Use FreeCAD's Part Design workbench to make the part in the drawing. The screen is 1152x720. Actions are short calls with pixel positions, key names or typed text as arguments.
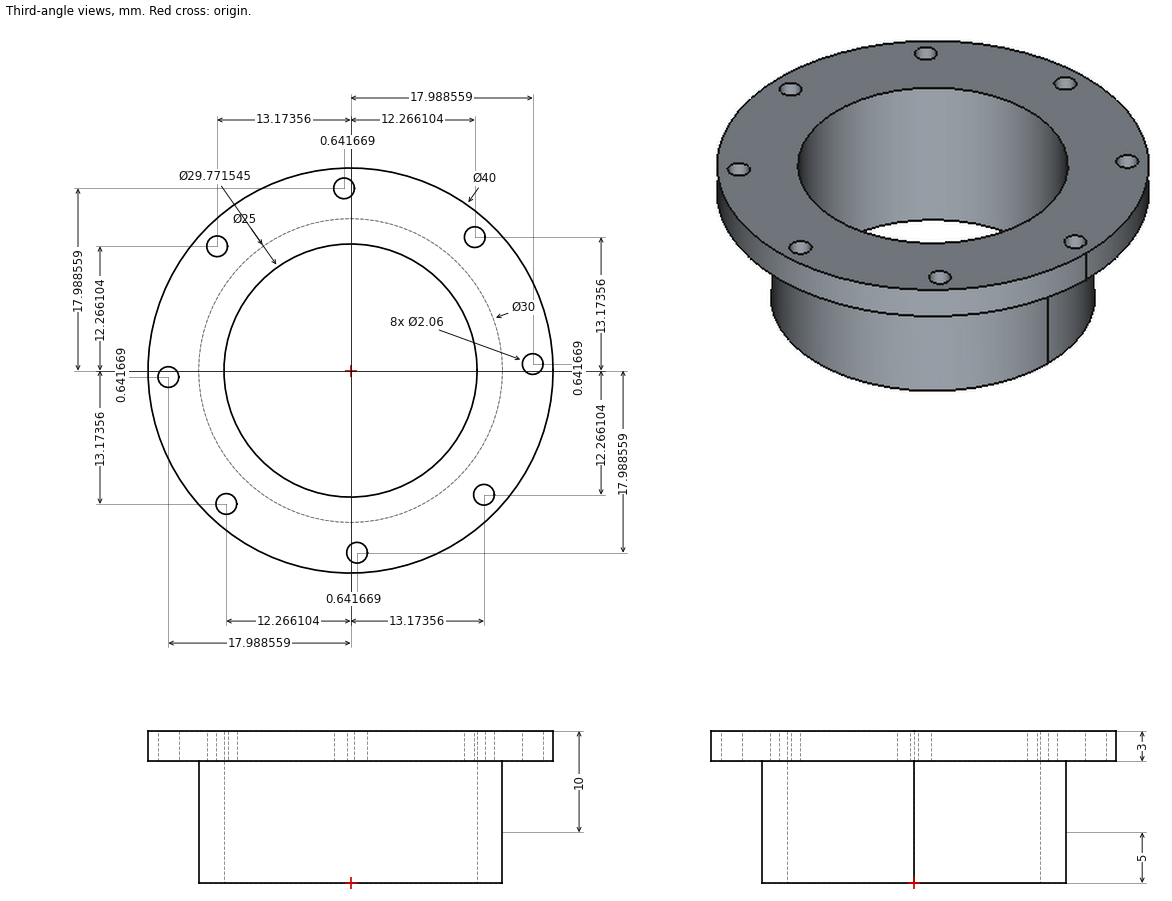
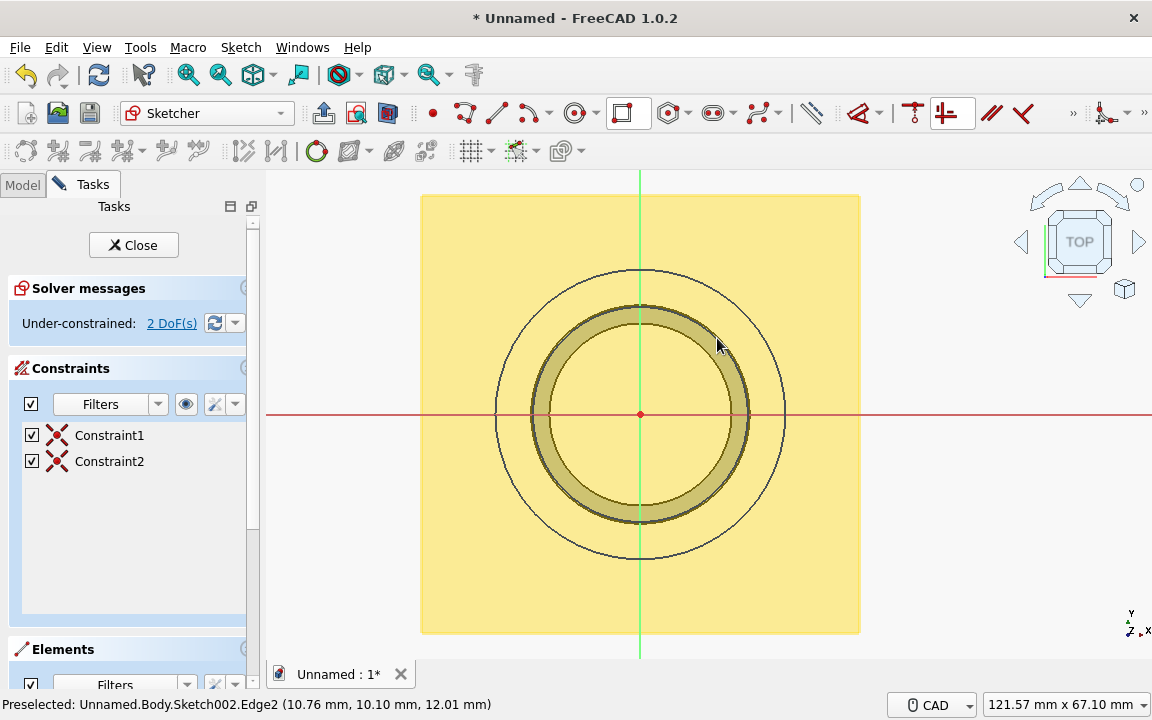
click(858, 114)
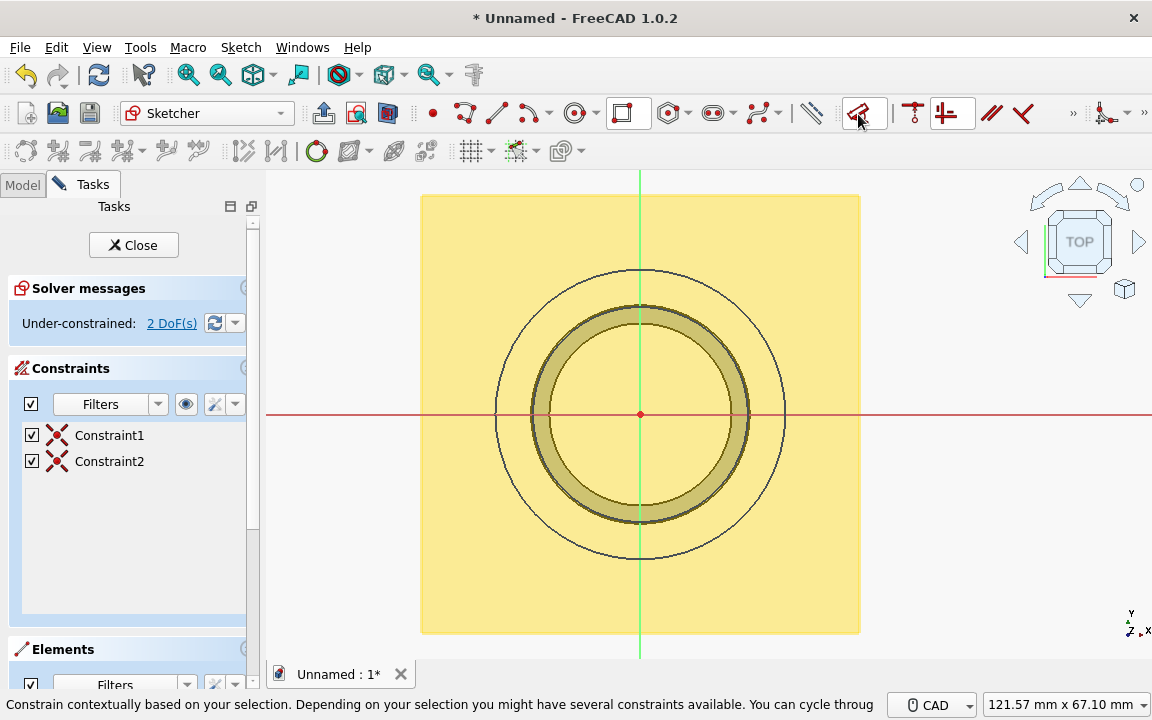
click(743, 312)
click(766, 289)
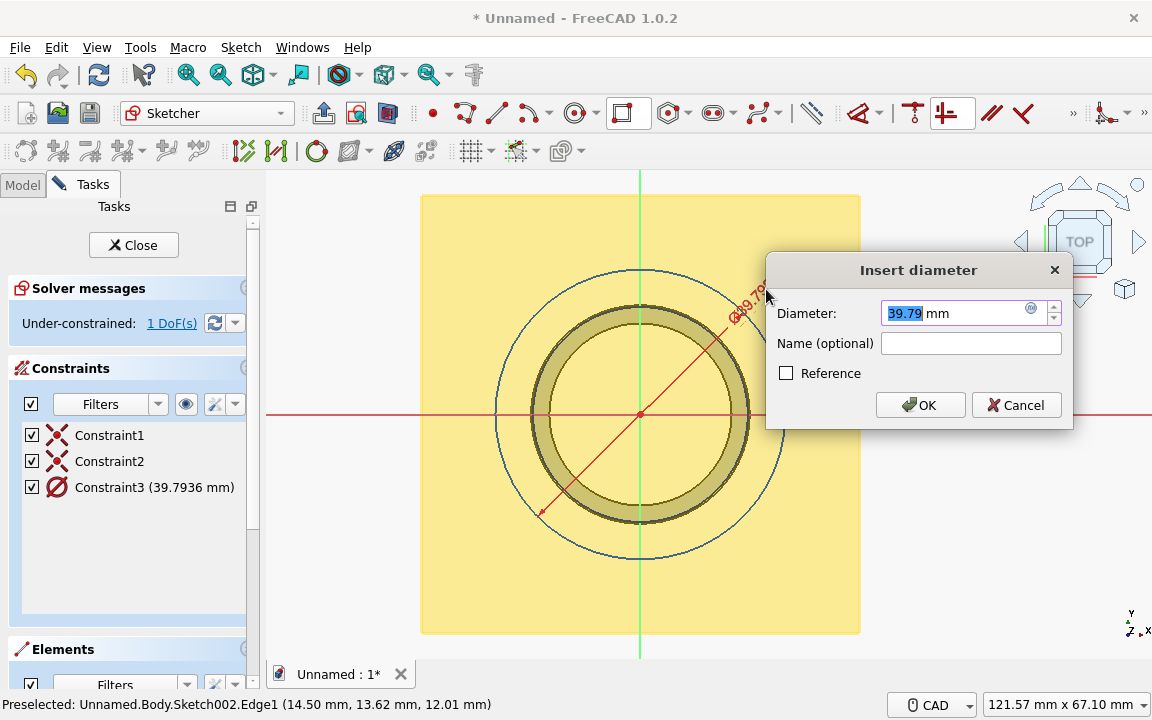
text(40)
key(Return)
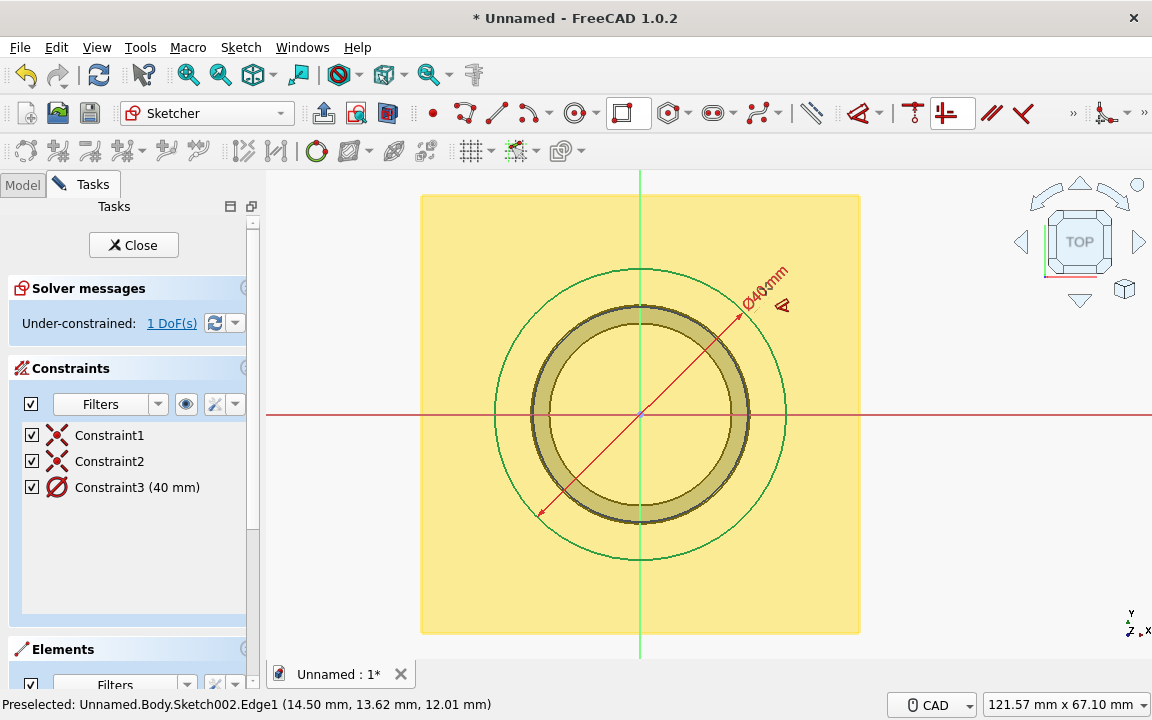
click(716, 338)
click(796, 368)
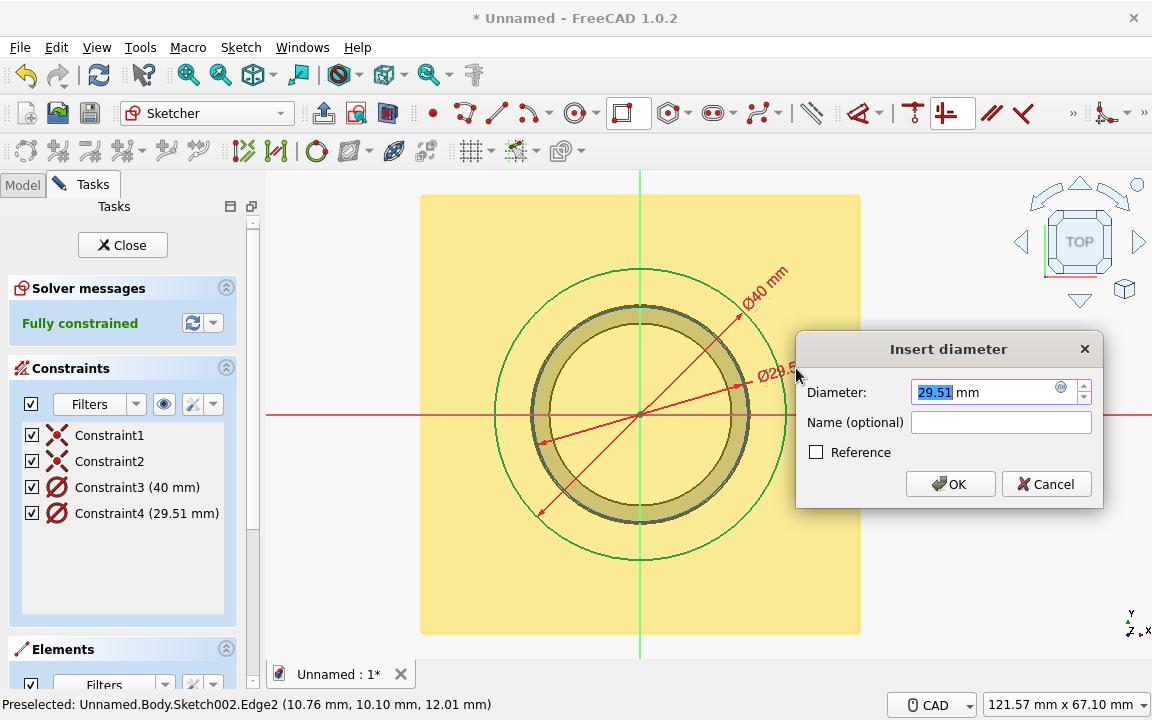
text(29.771545)
key(Return)
key(Escape)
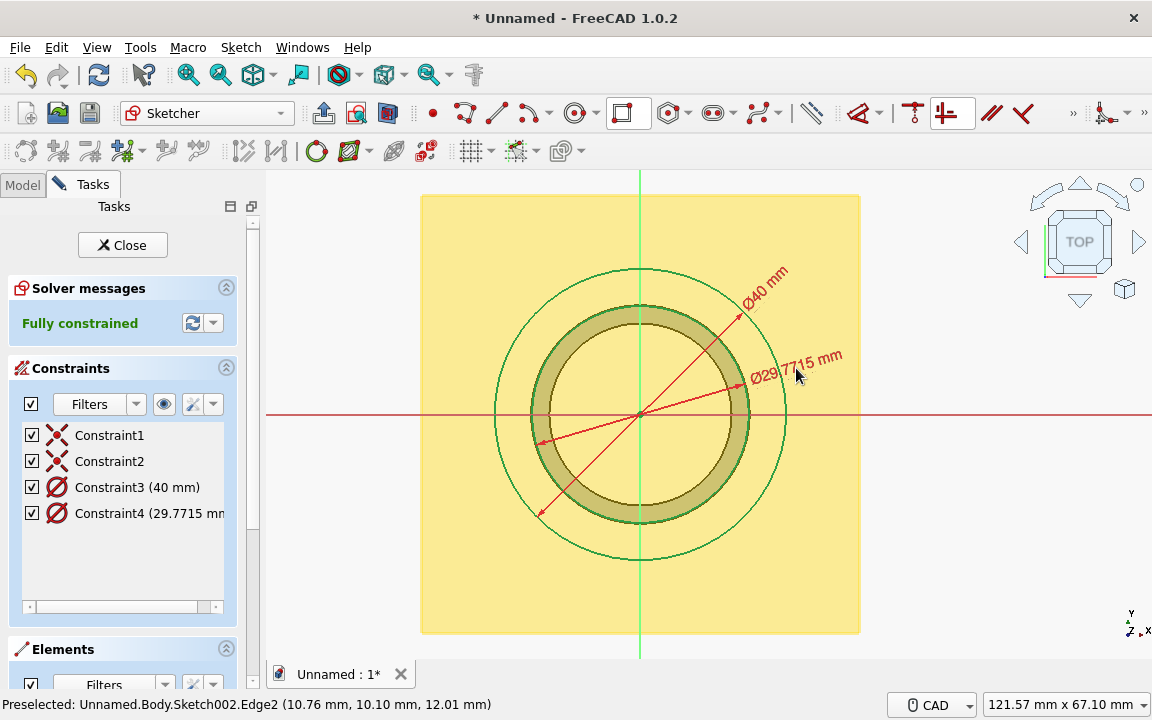
click(123, 245)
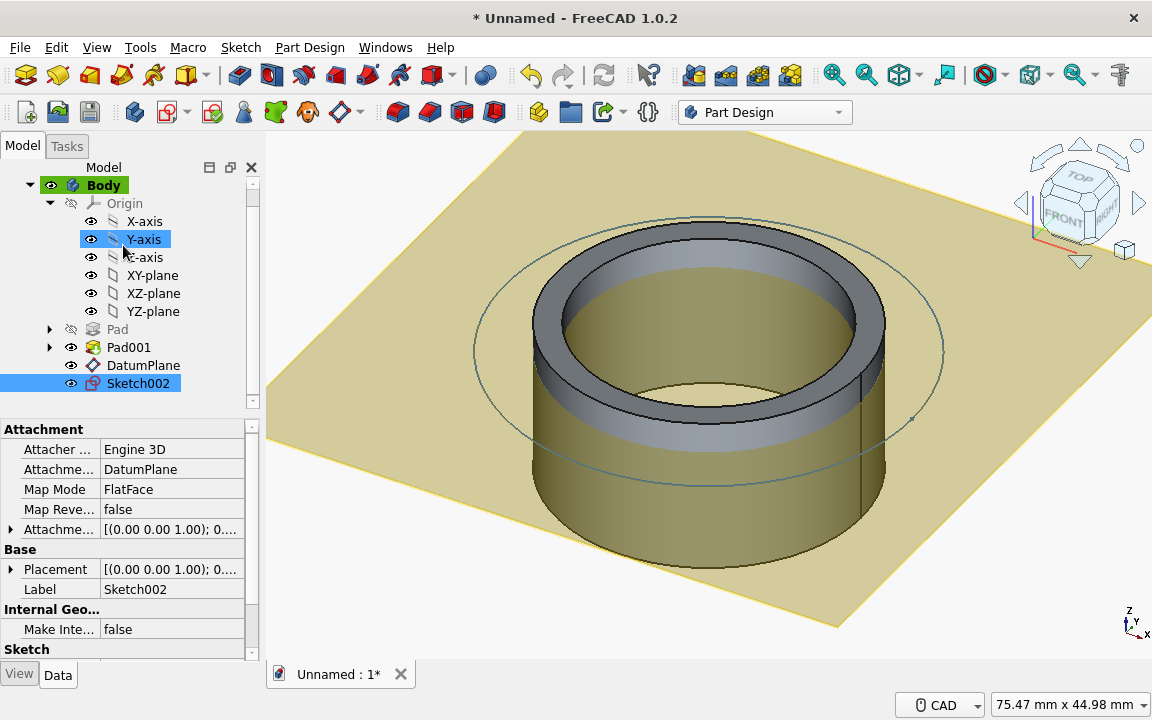
click(26, 76)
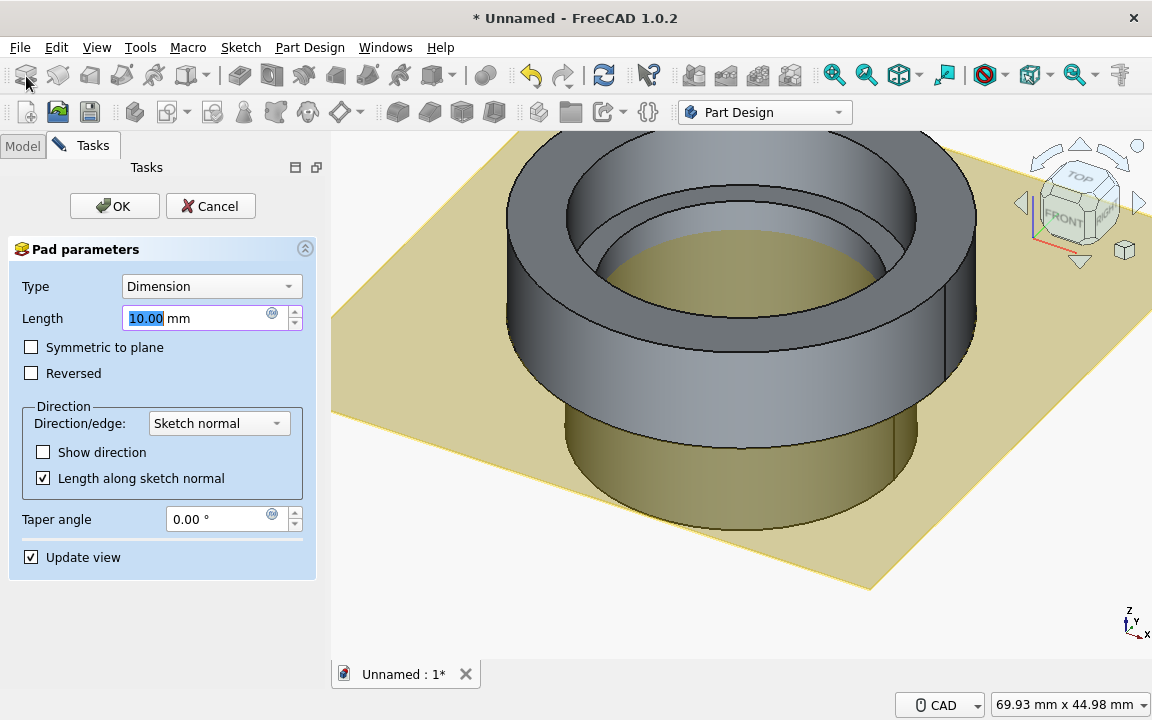
text(3)
key(Tab)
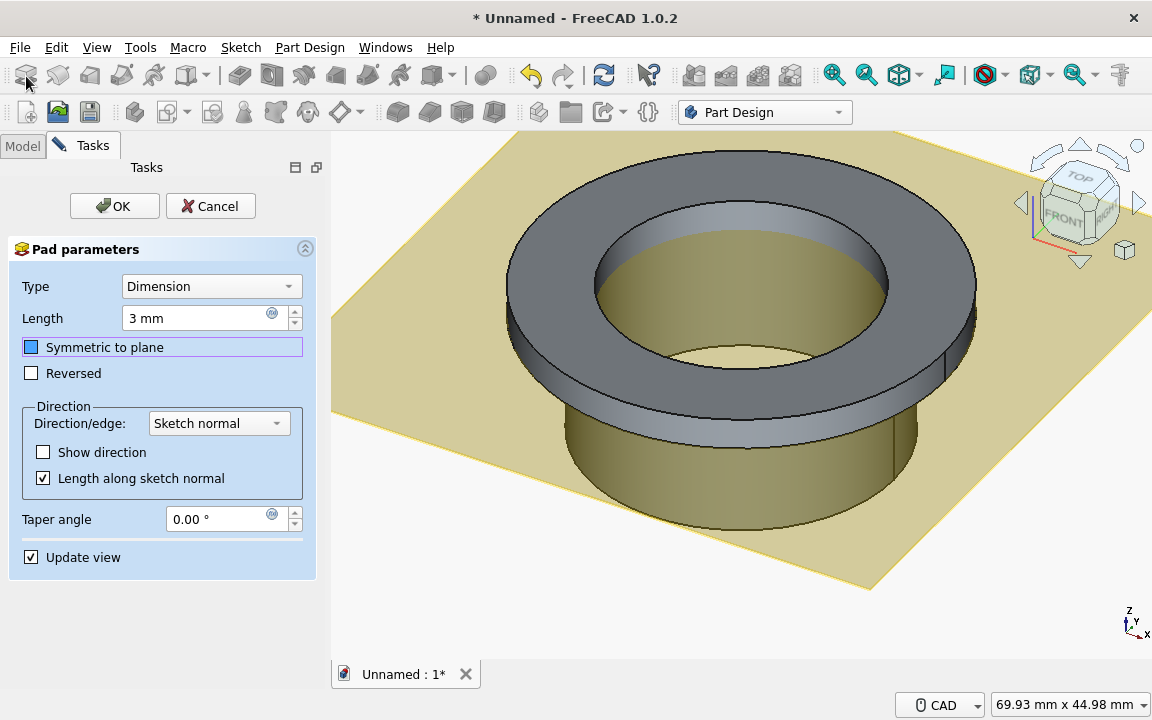
click(115, 206)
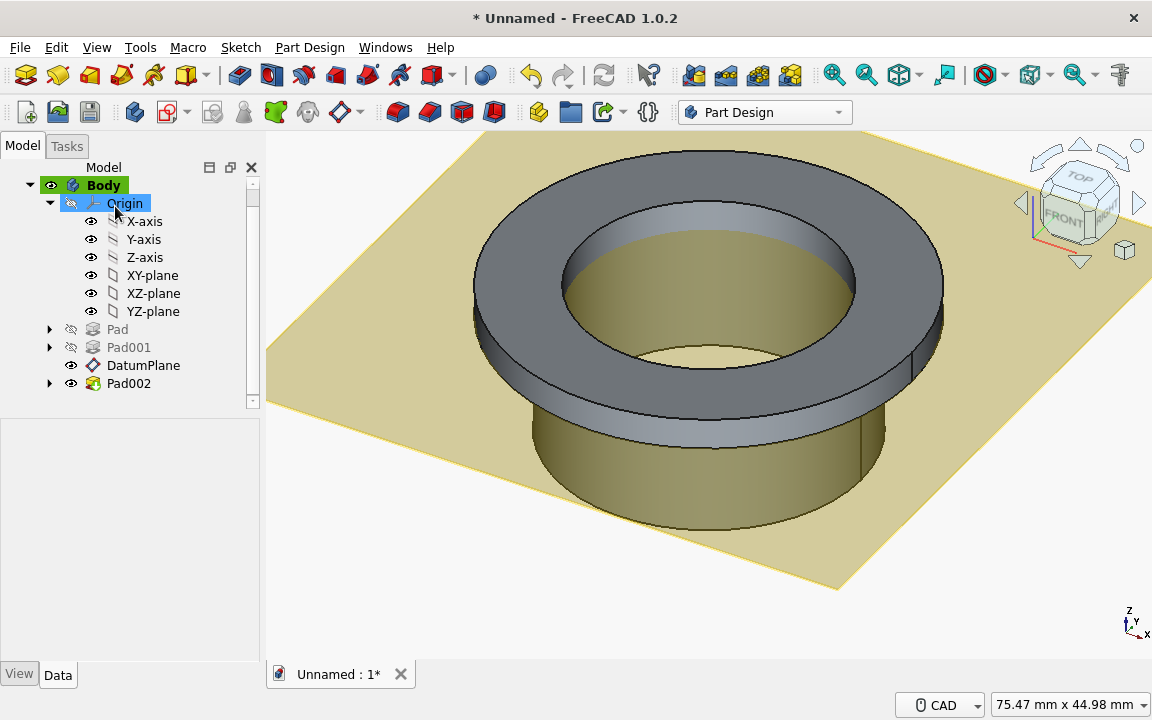
click(116, 365)
key(space)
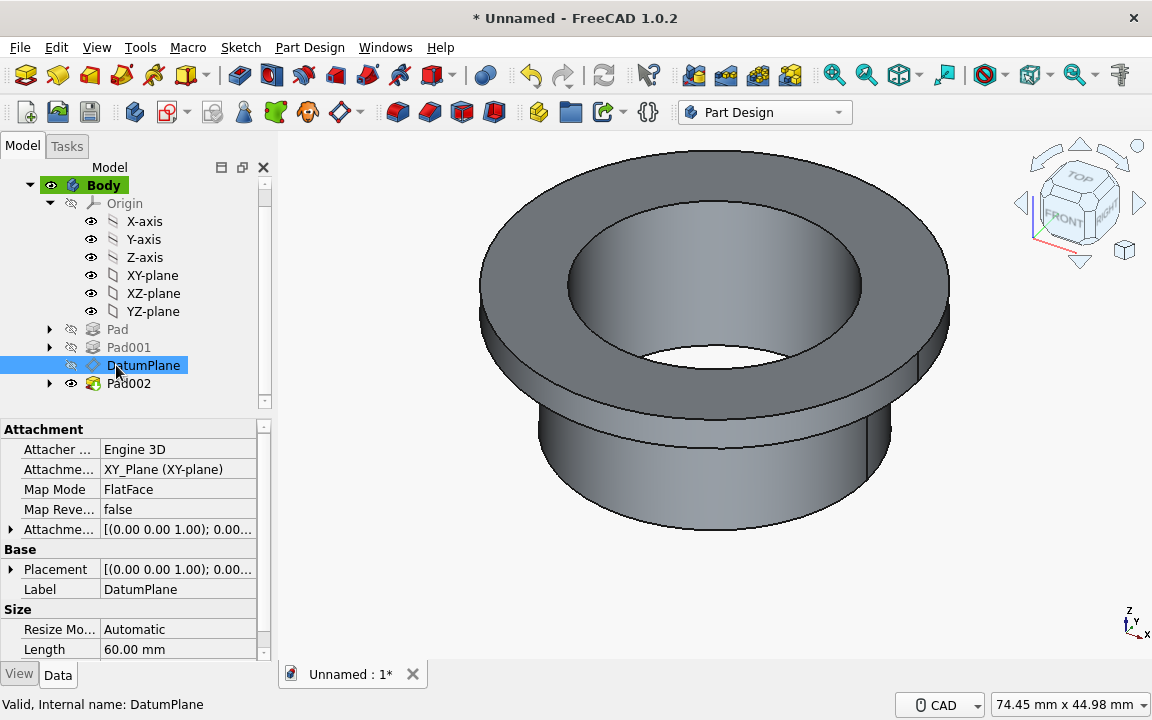
key(v)
key(f)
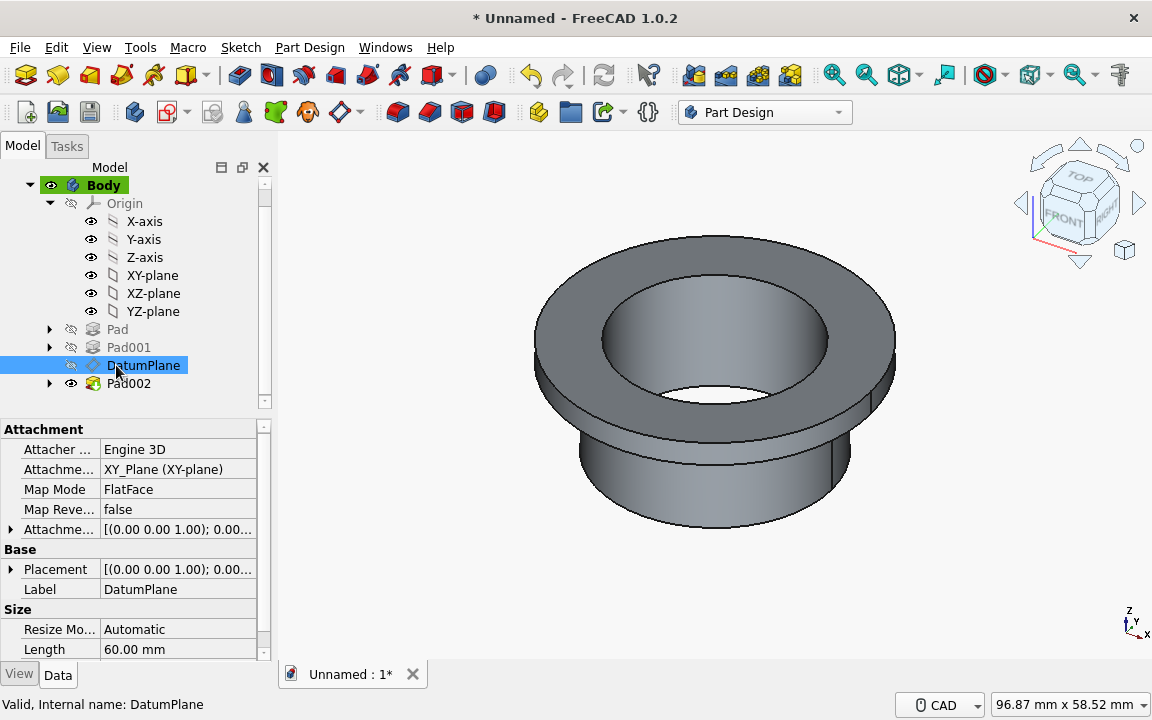
click(677, 258)